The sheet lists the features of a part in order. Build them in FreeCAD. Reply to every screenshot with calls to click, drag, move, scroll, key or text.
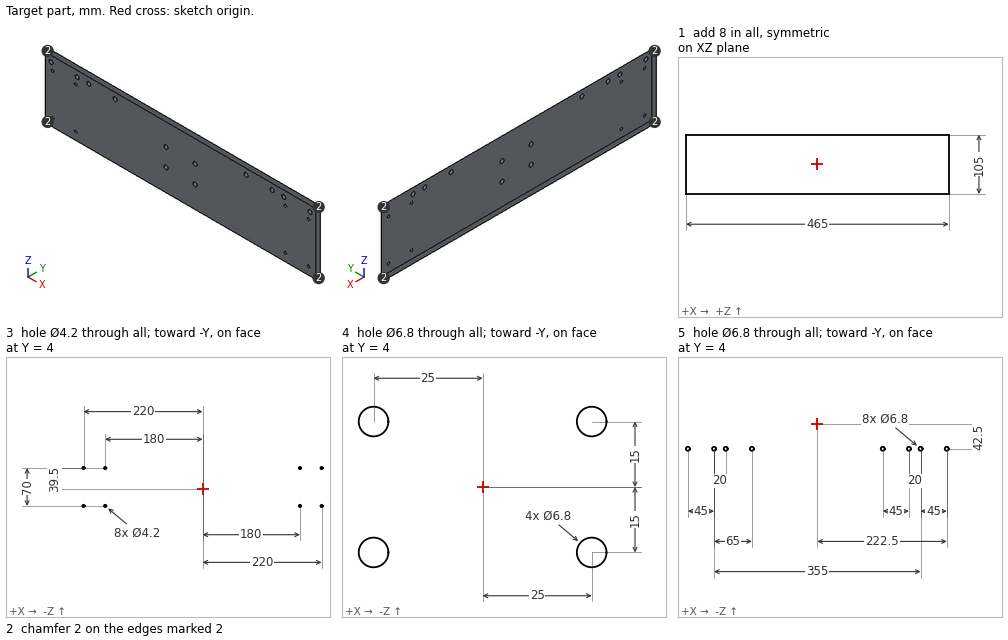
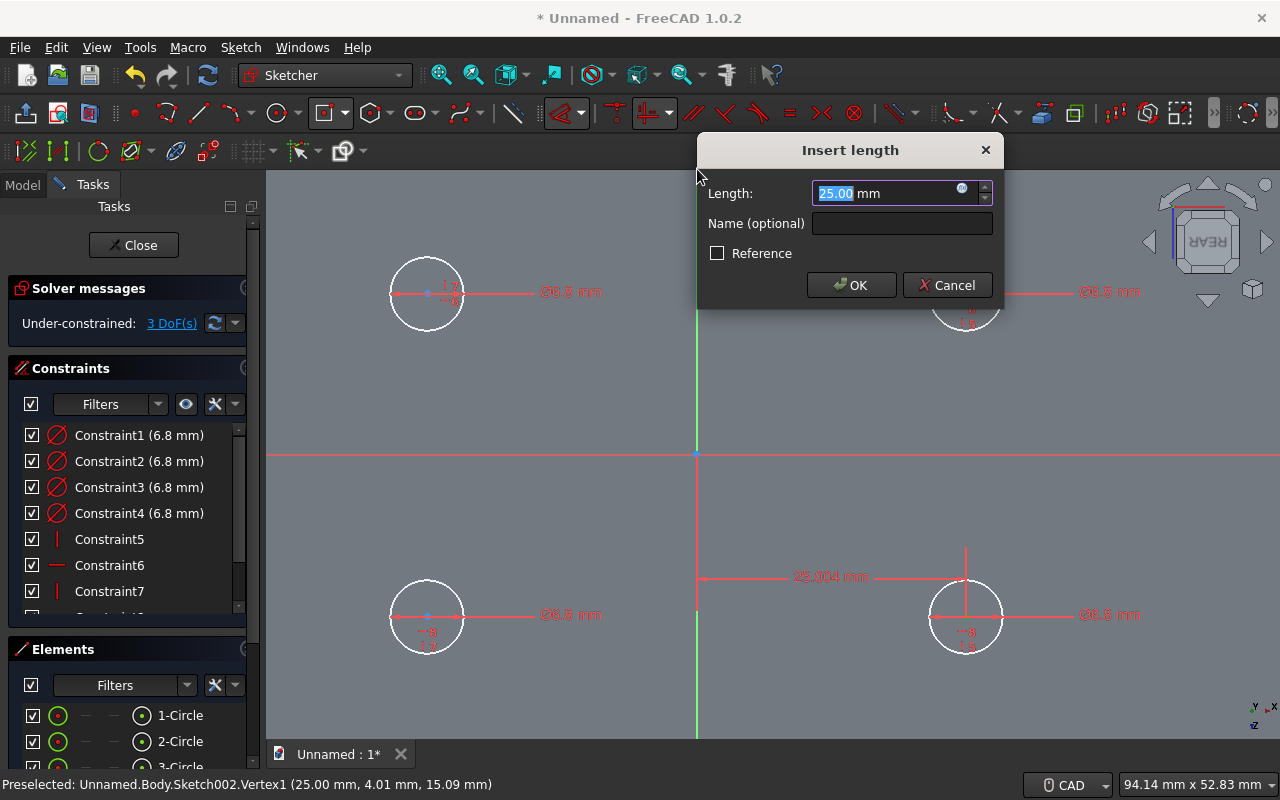
text(25)
key(Return)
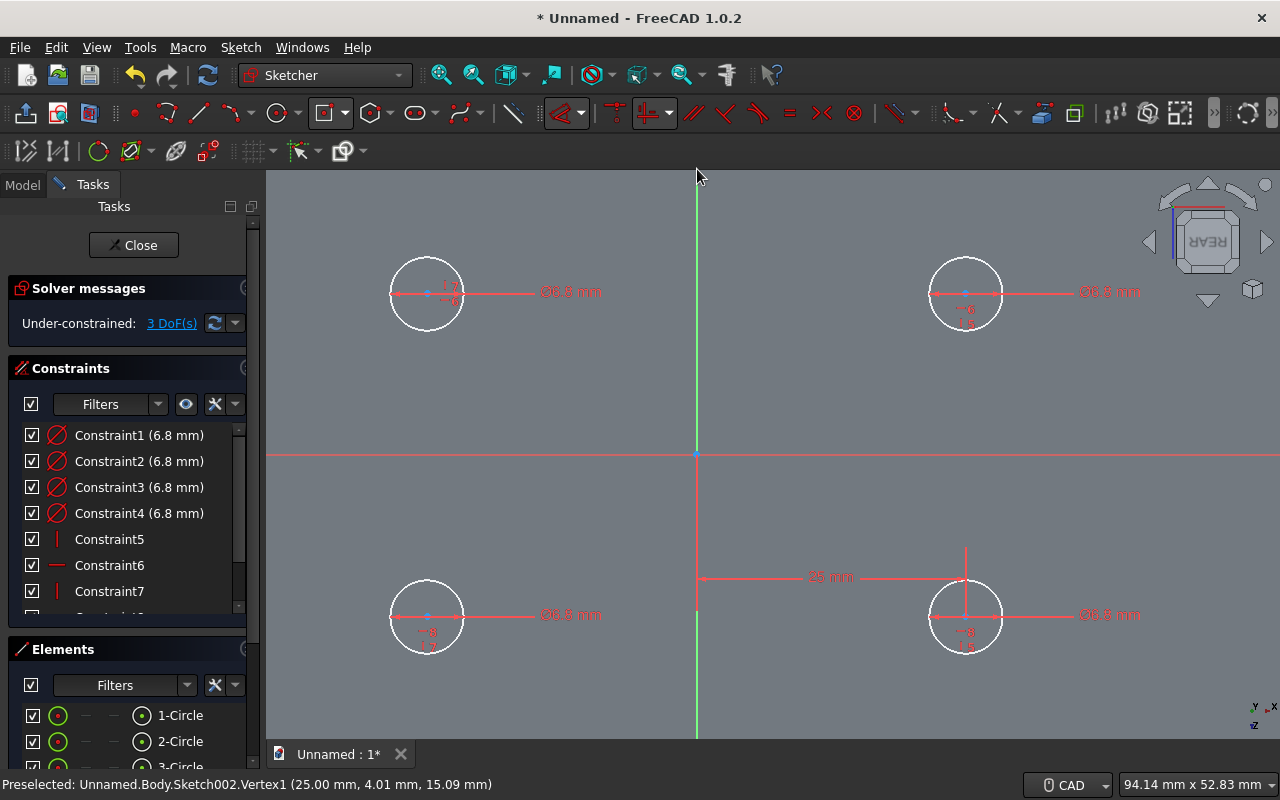
click(966, 617)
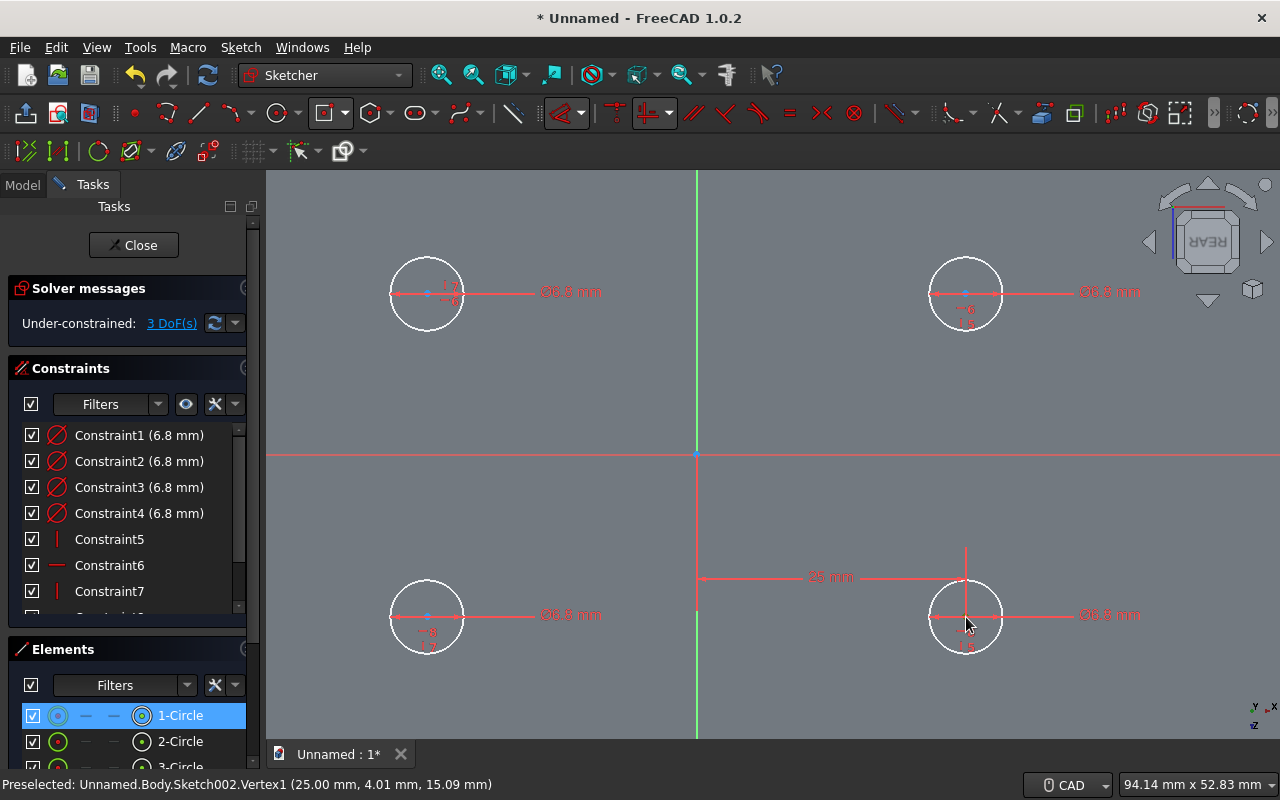
key(i)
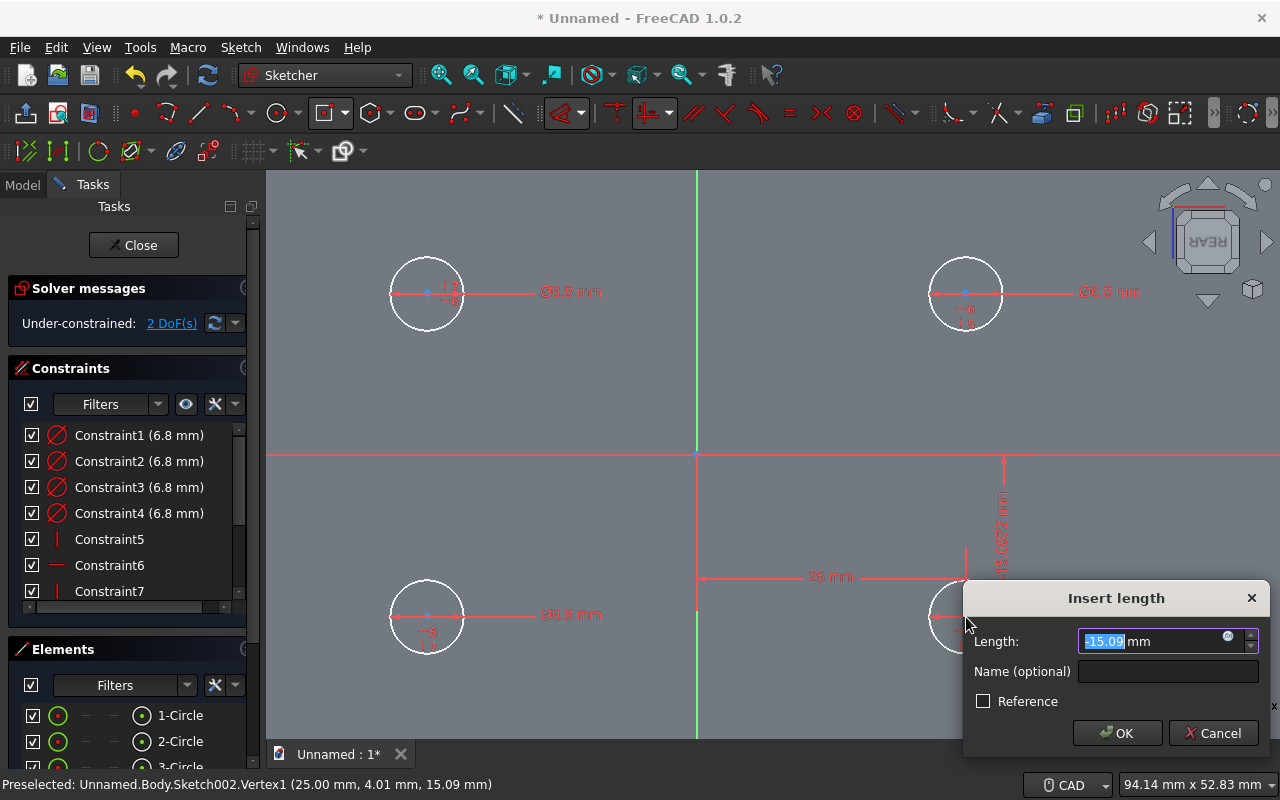
text(-15)
key(Return)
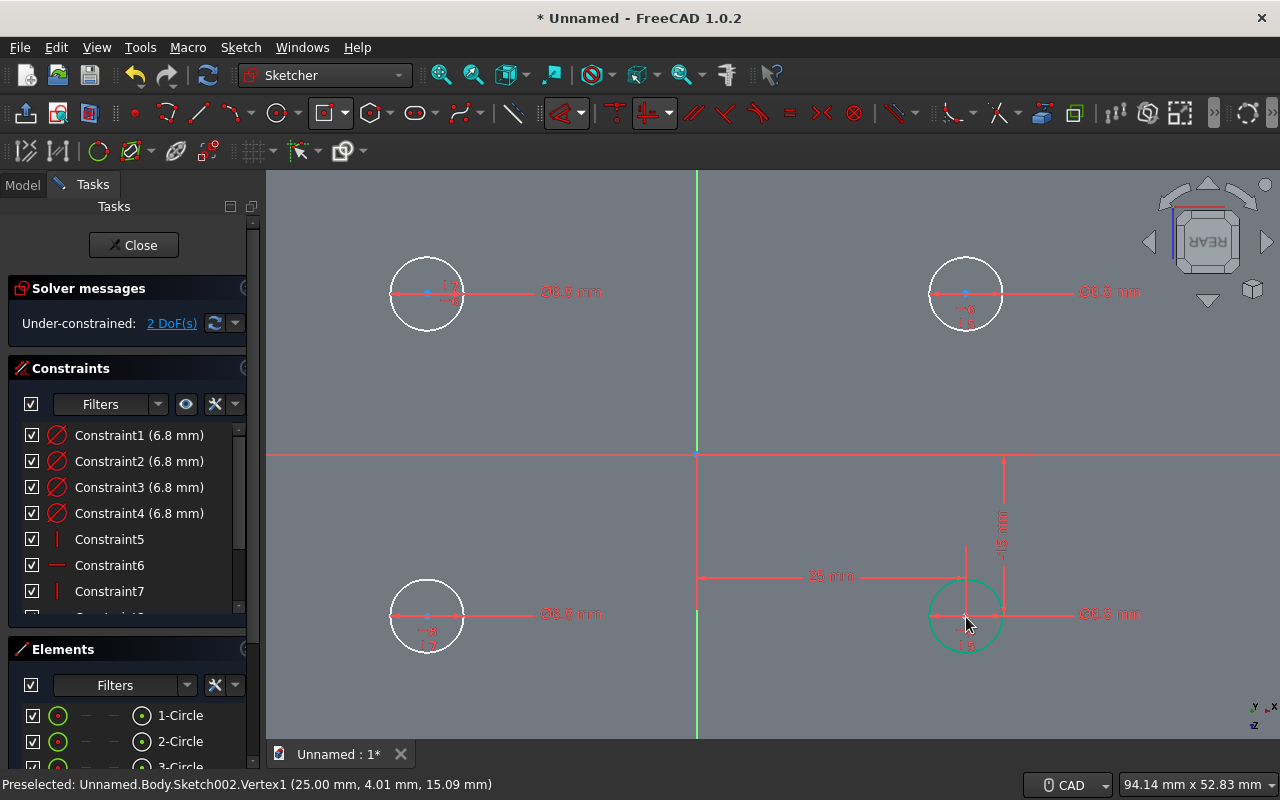
click(966, 294)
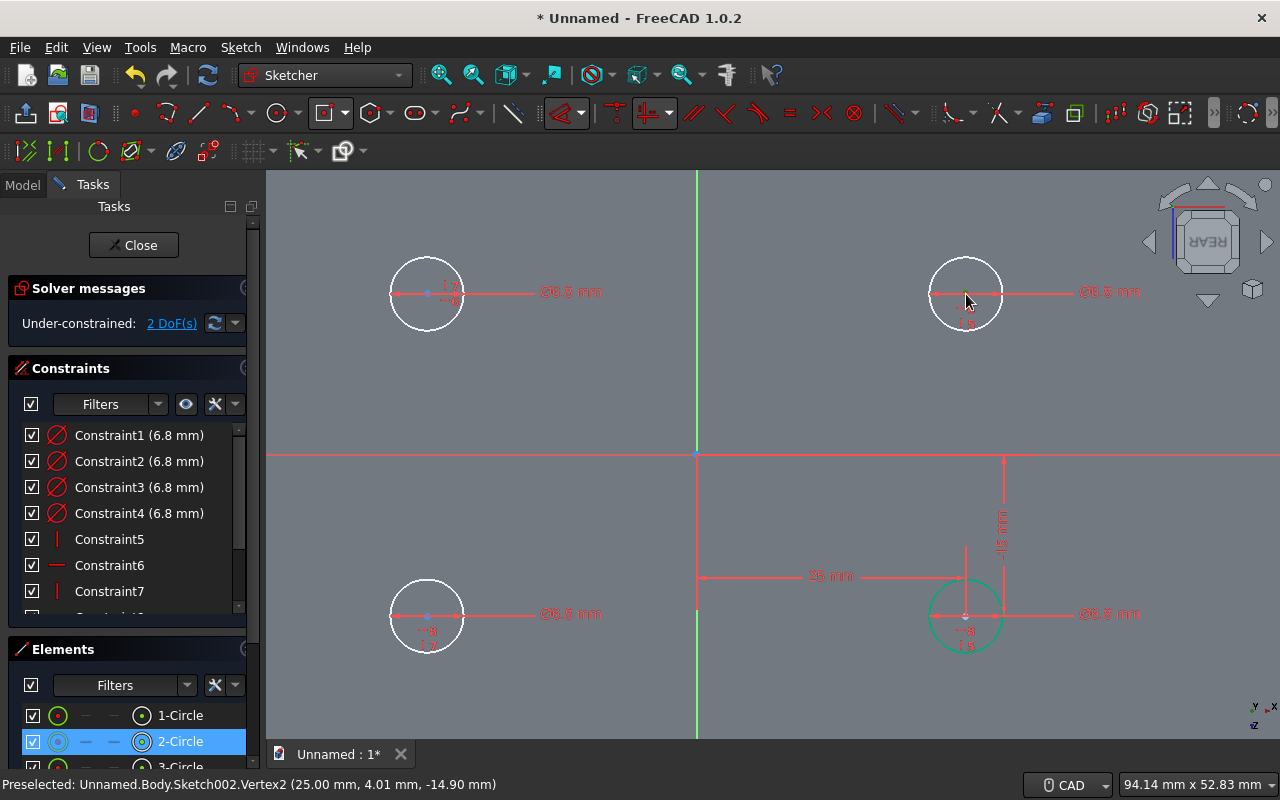
click(584, 114)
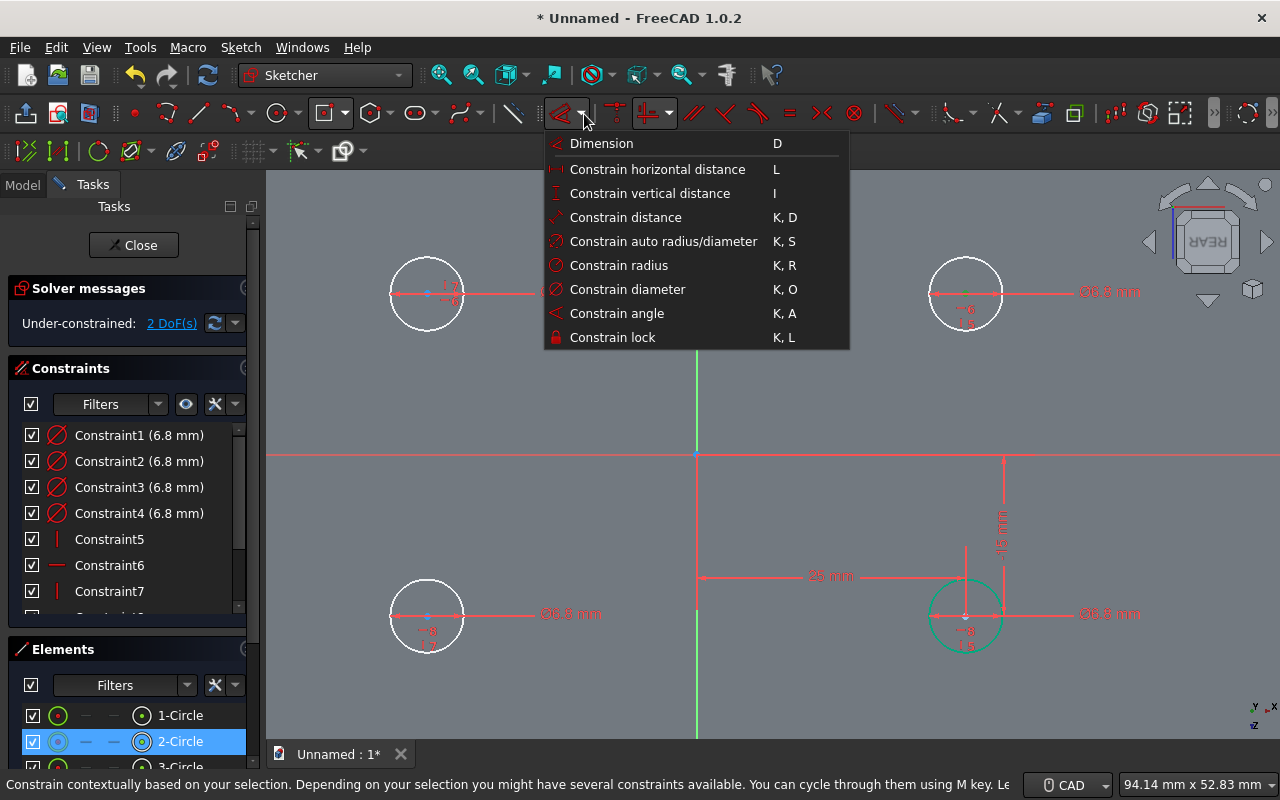
click(697, 193)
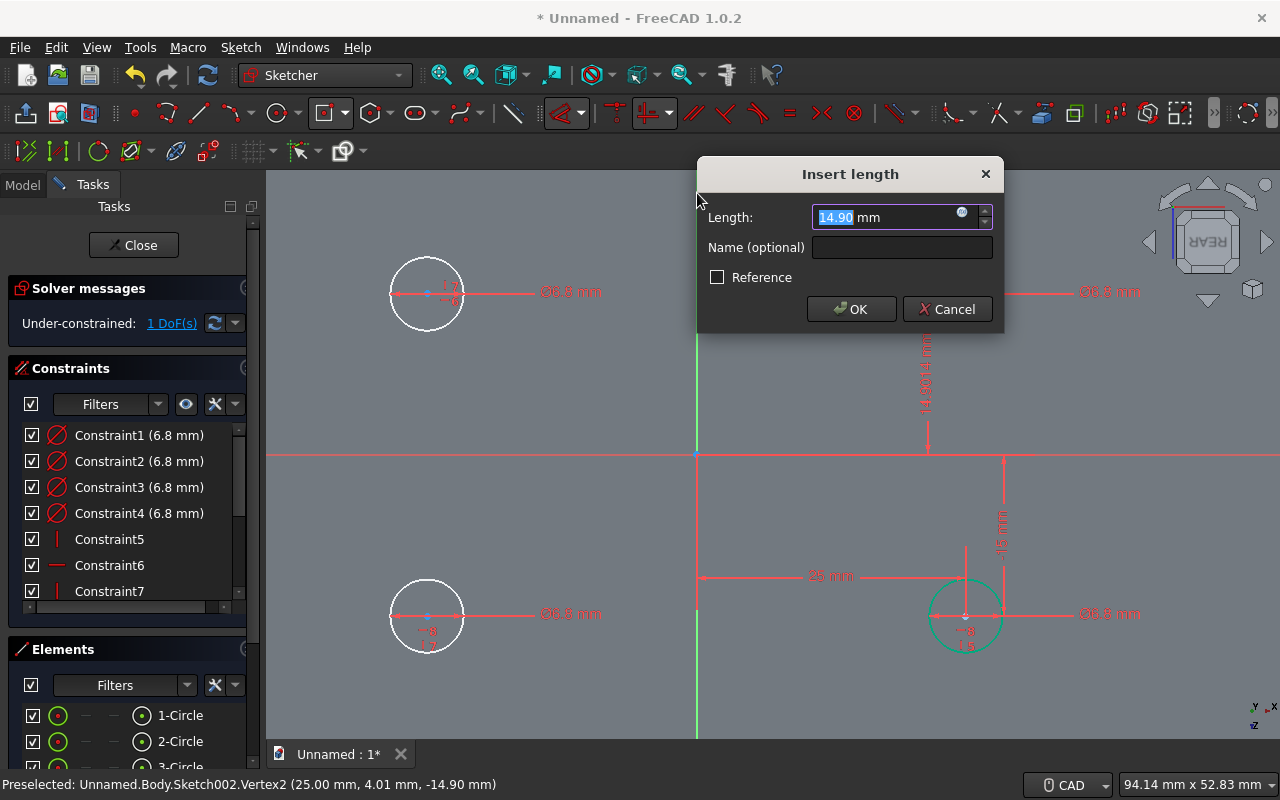
text(15)
key(Return)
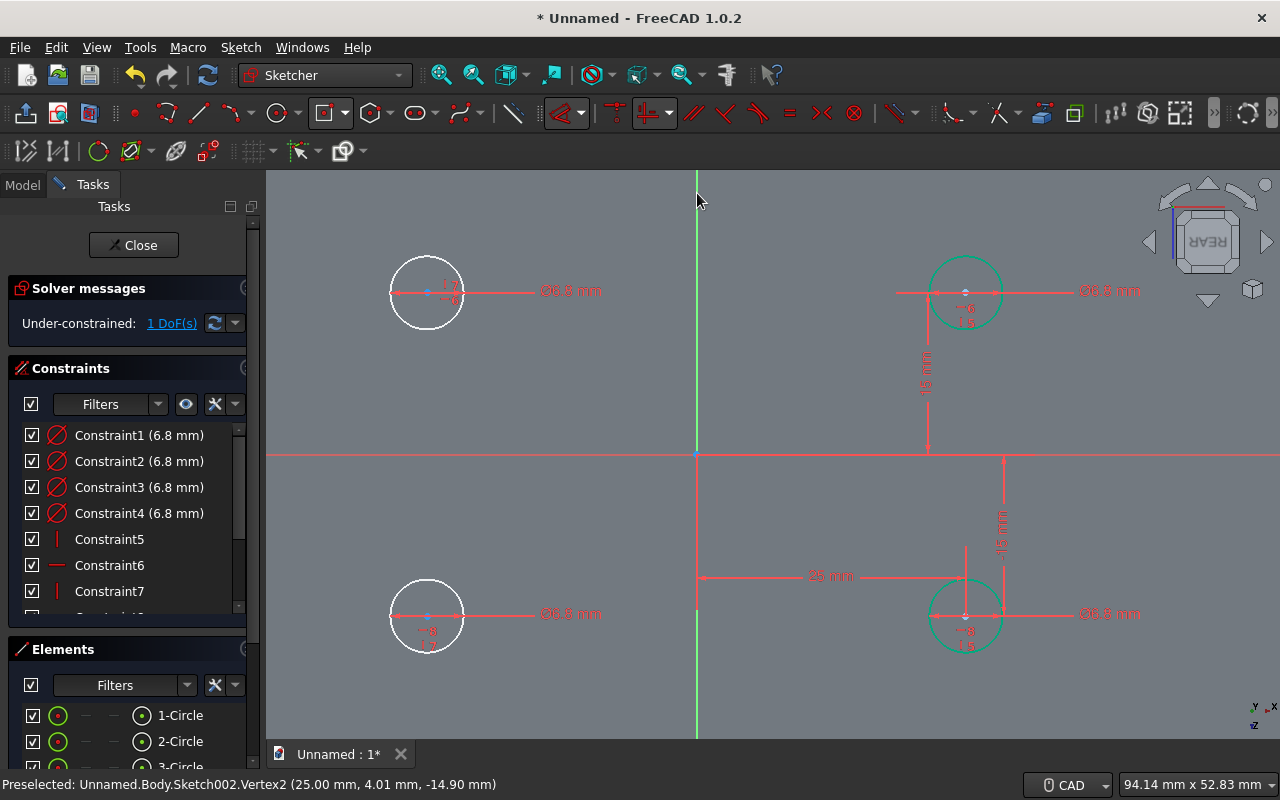
click(427, 293)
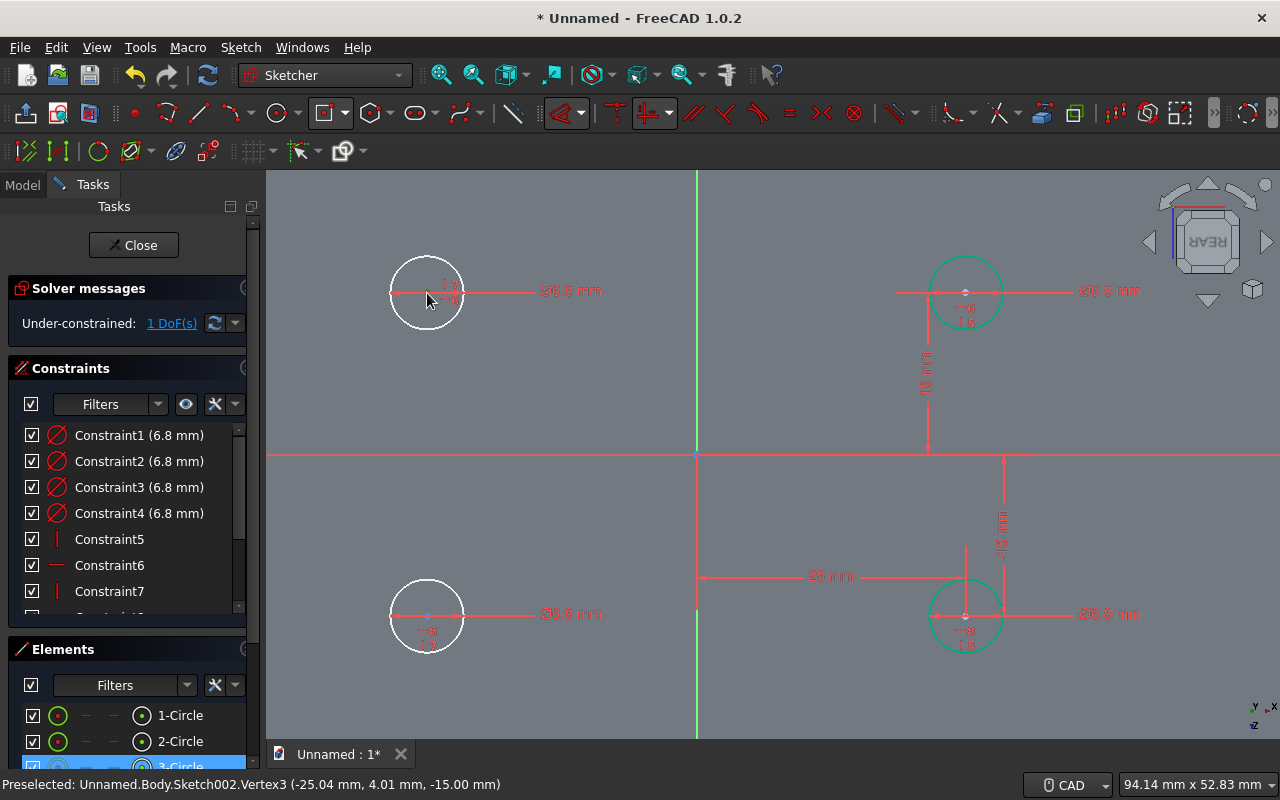
key(l)